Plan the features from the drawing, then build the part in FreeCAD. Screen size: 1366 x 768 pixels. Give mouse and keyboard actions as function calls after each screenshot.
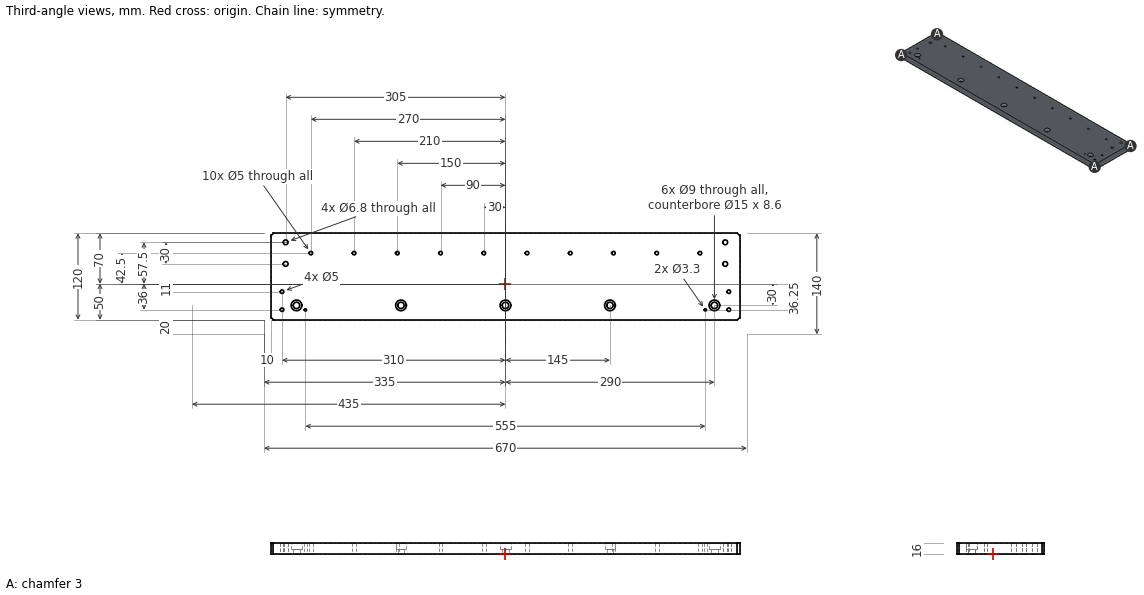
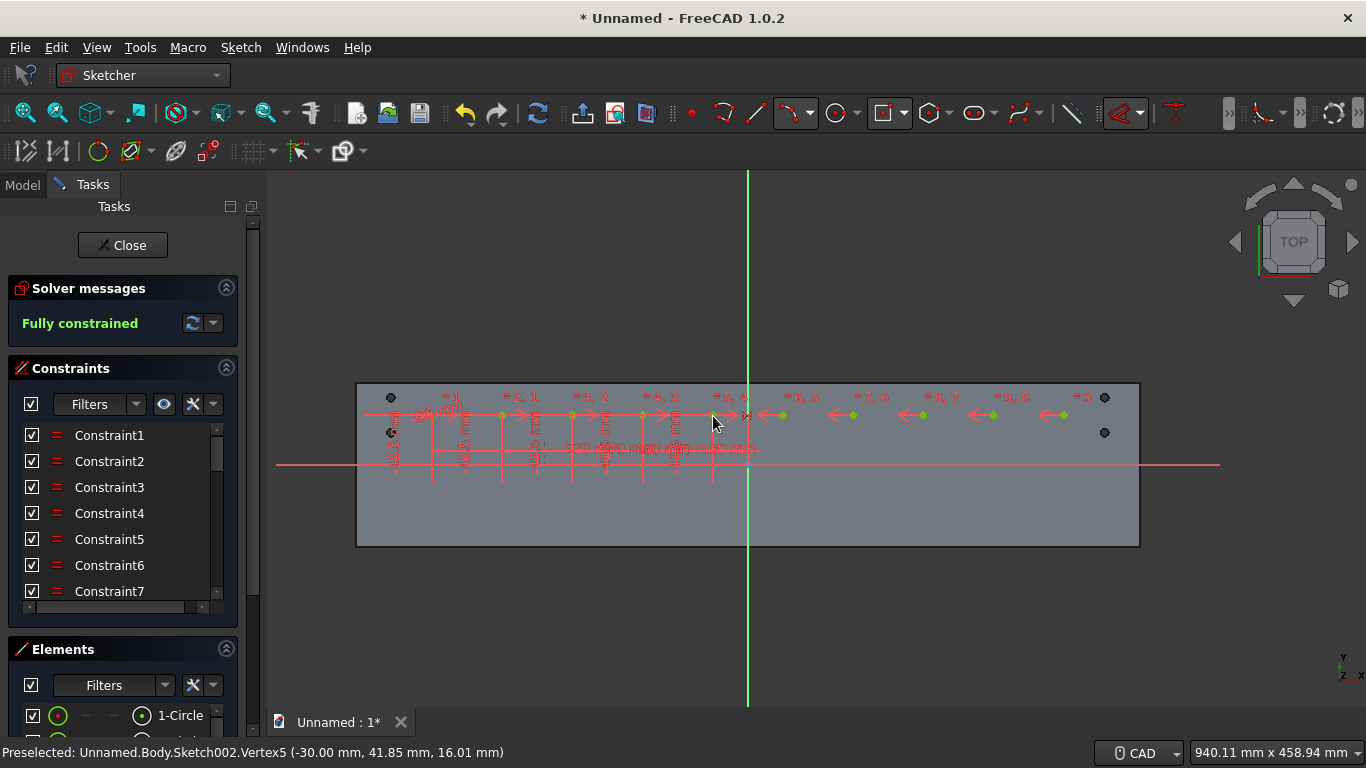
click(123, 245)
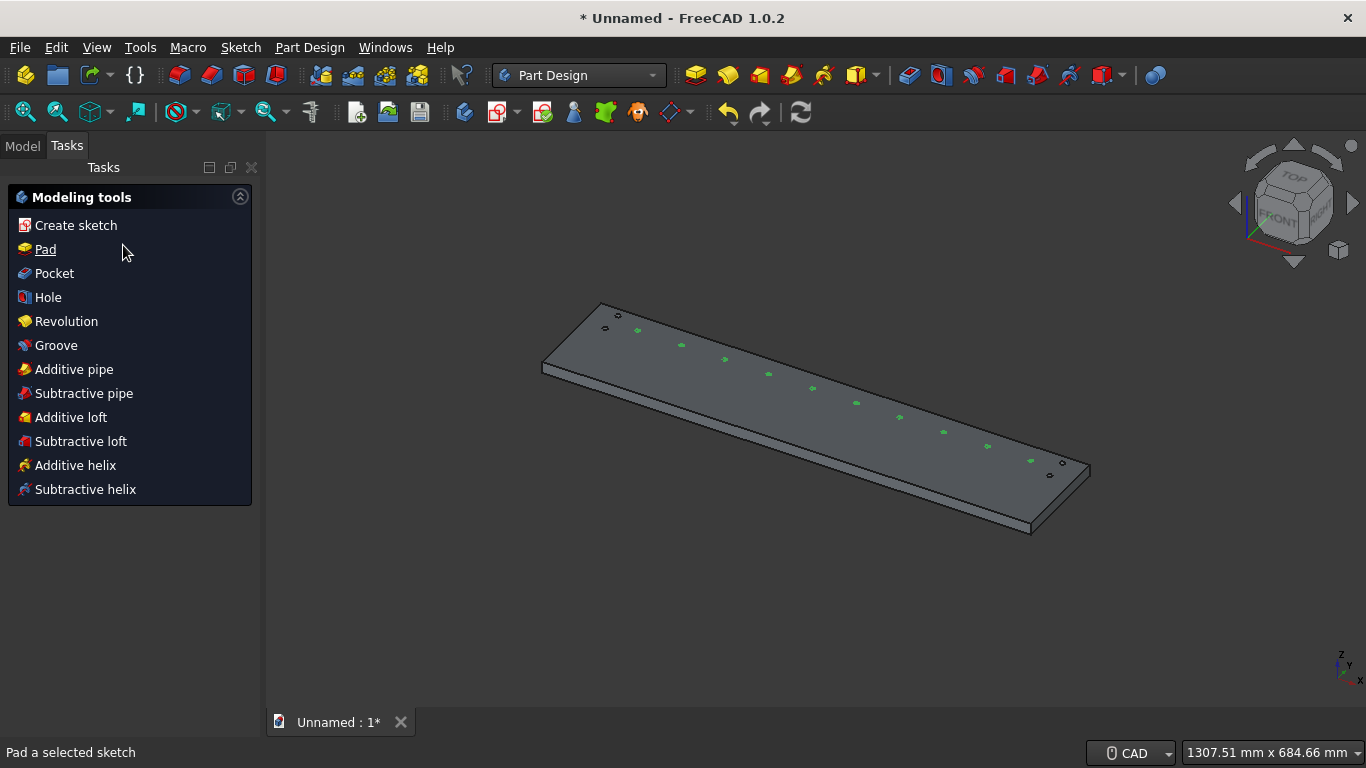
click(942, 76)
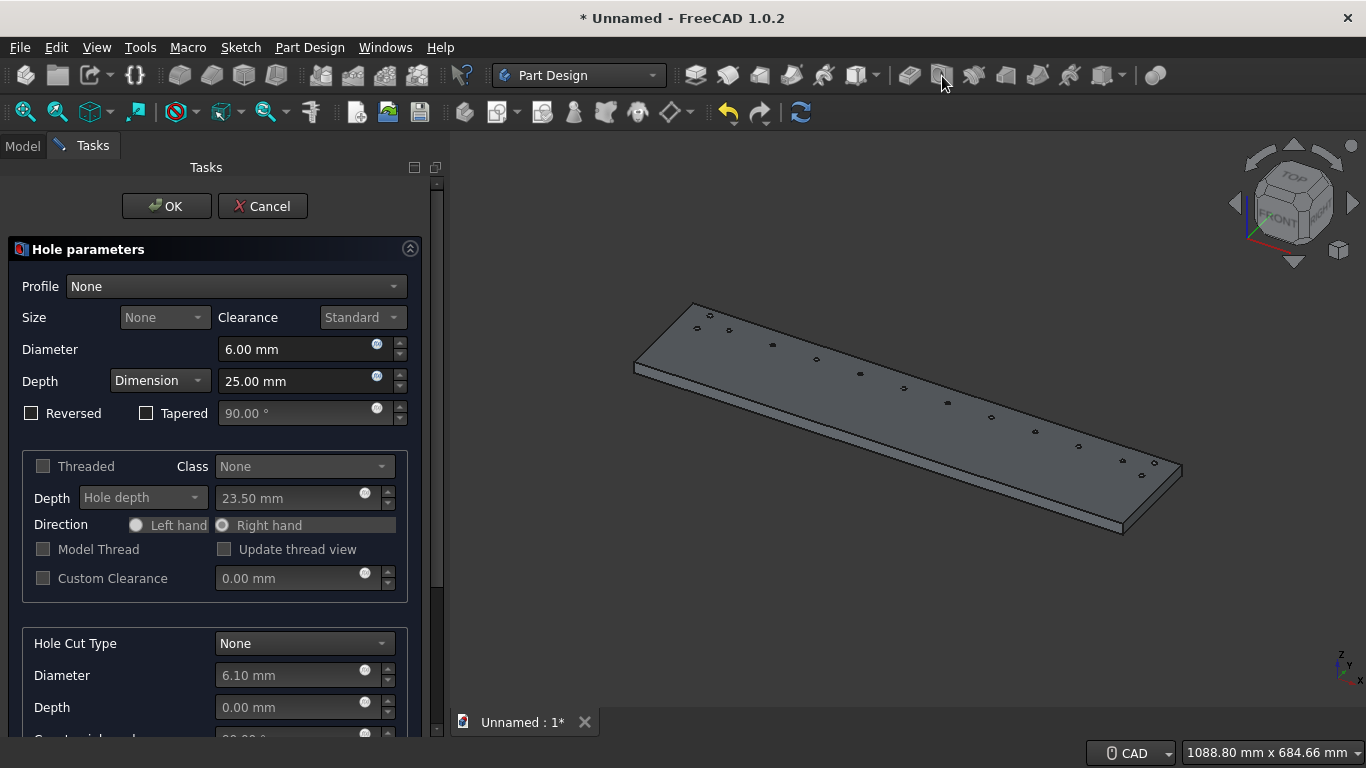
triple_click(305, 349)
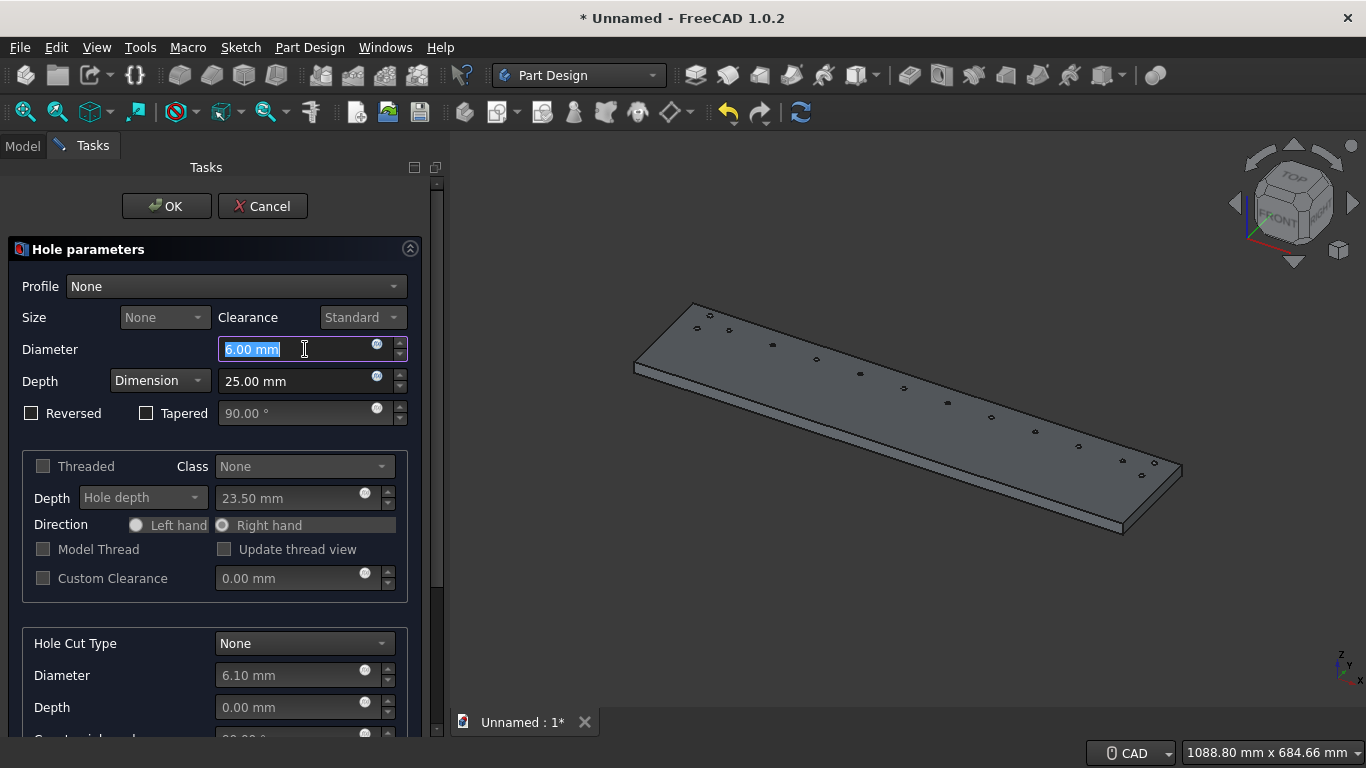
text(5)
key(Tab)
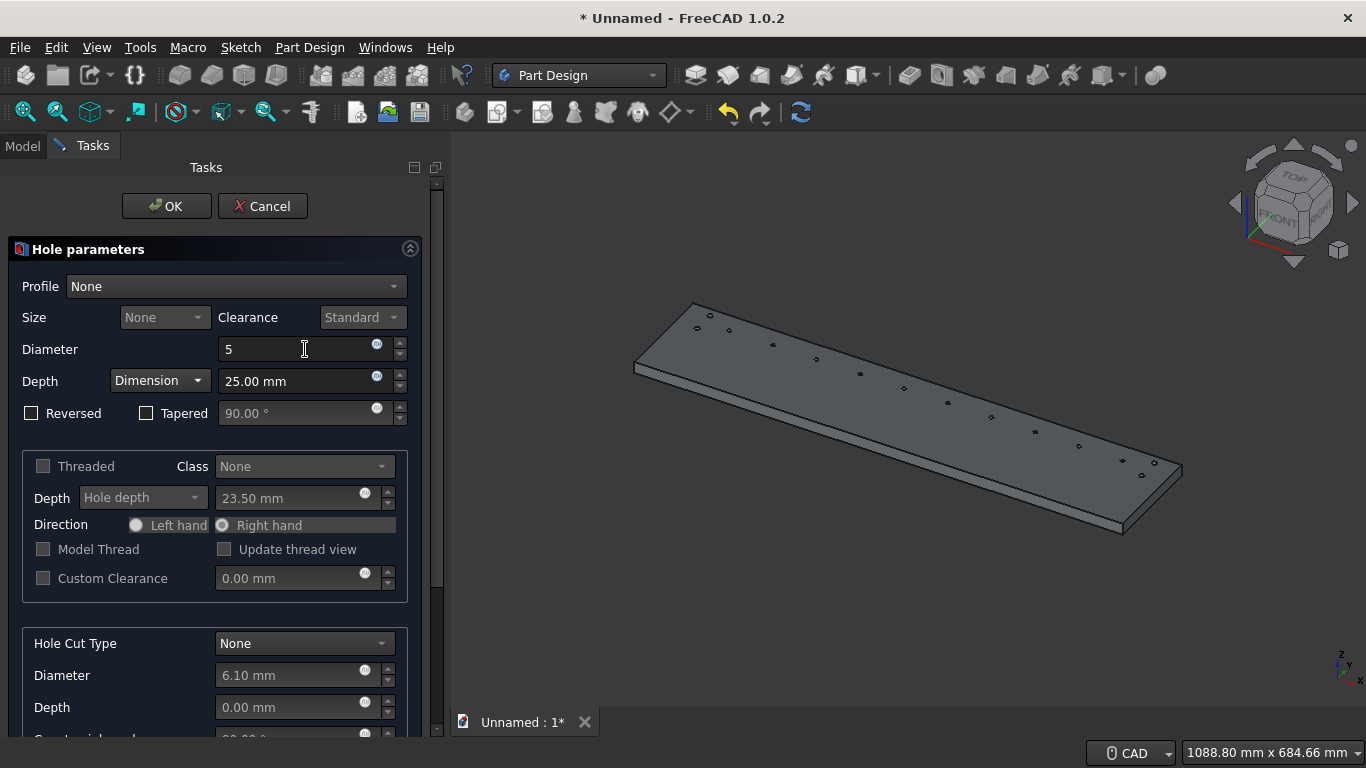
click(161, 380)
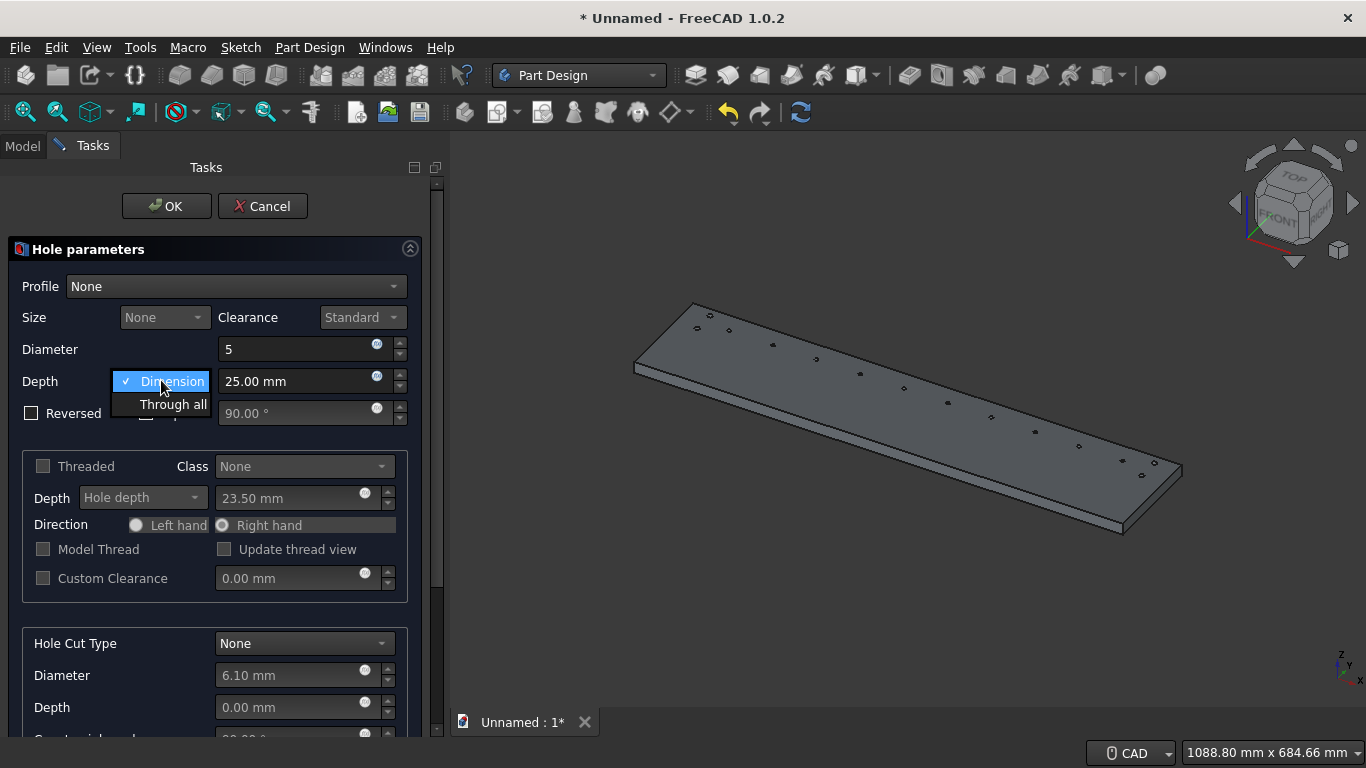
click(160, 404)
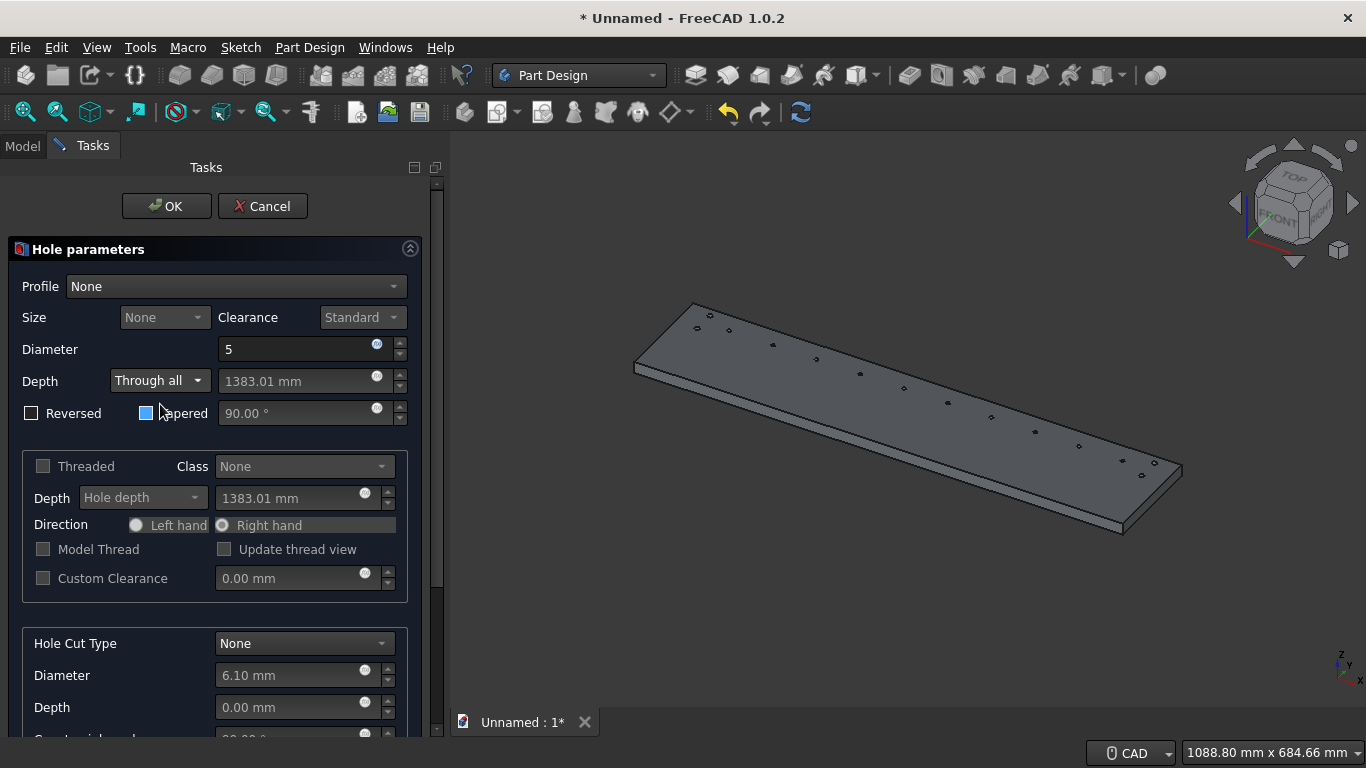
click(167, 206)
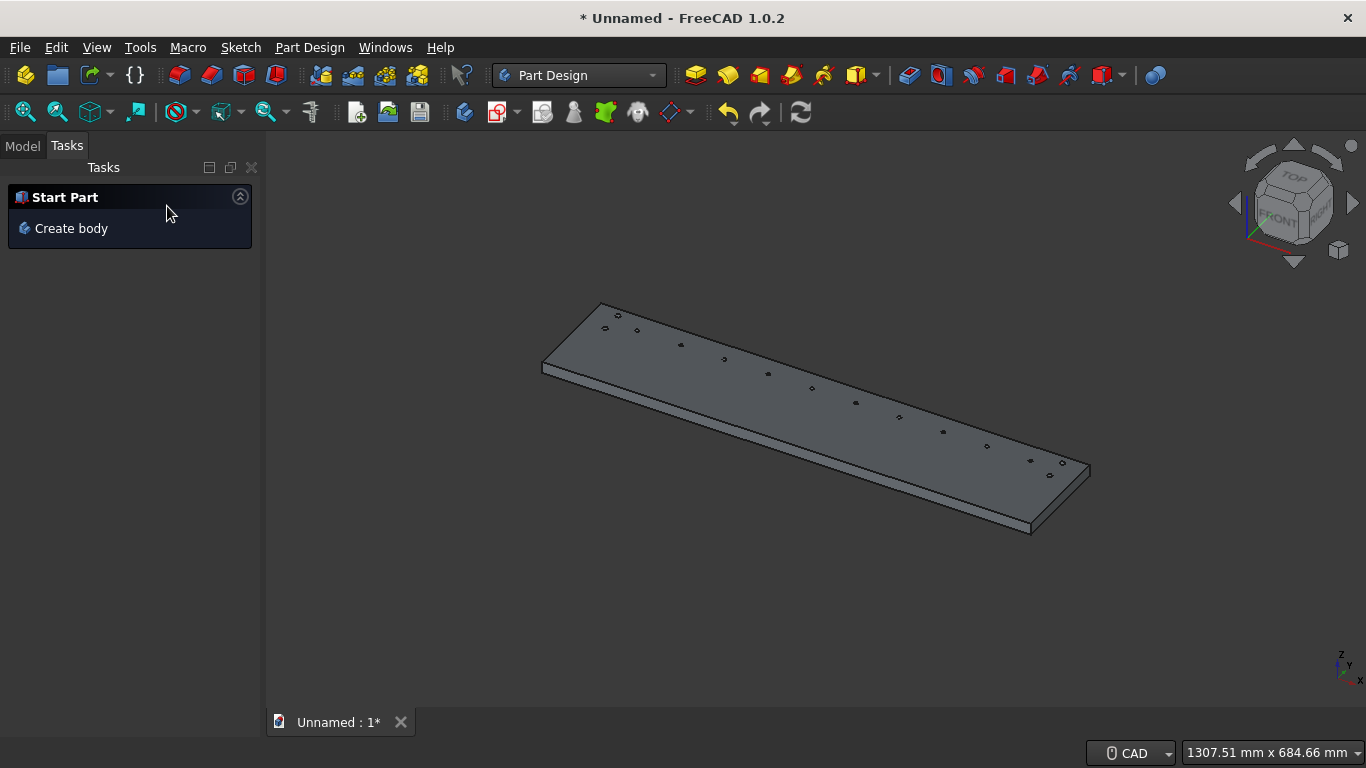
click(947, 467)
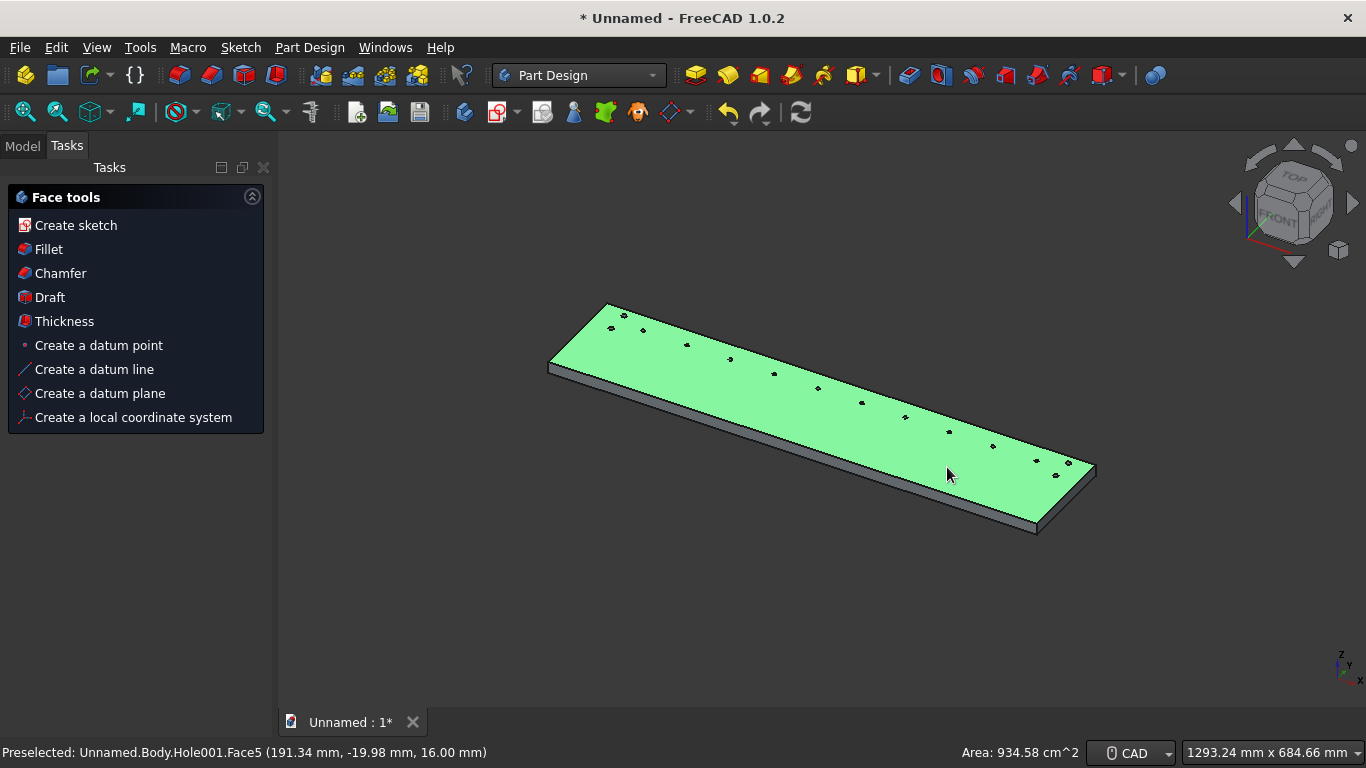
click(498, 112)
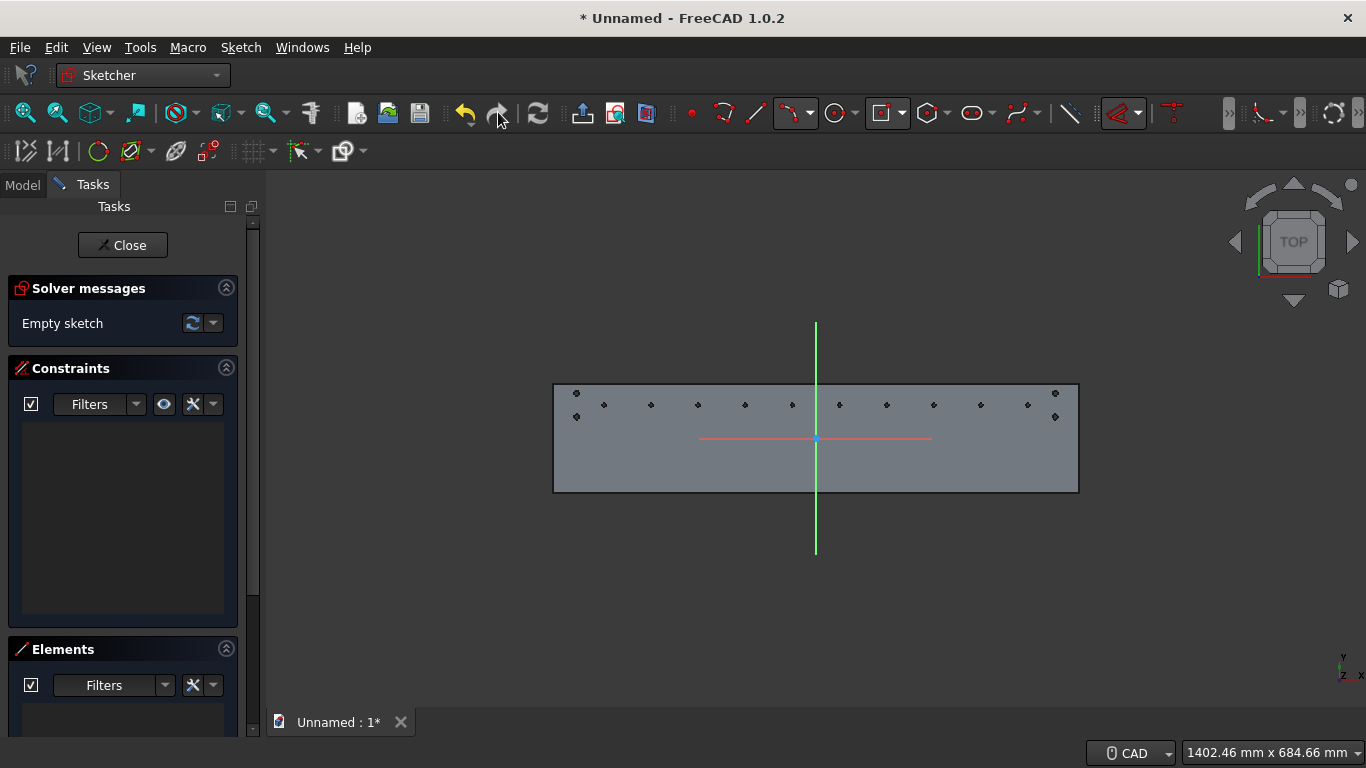
click(836, 114)